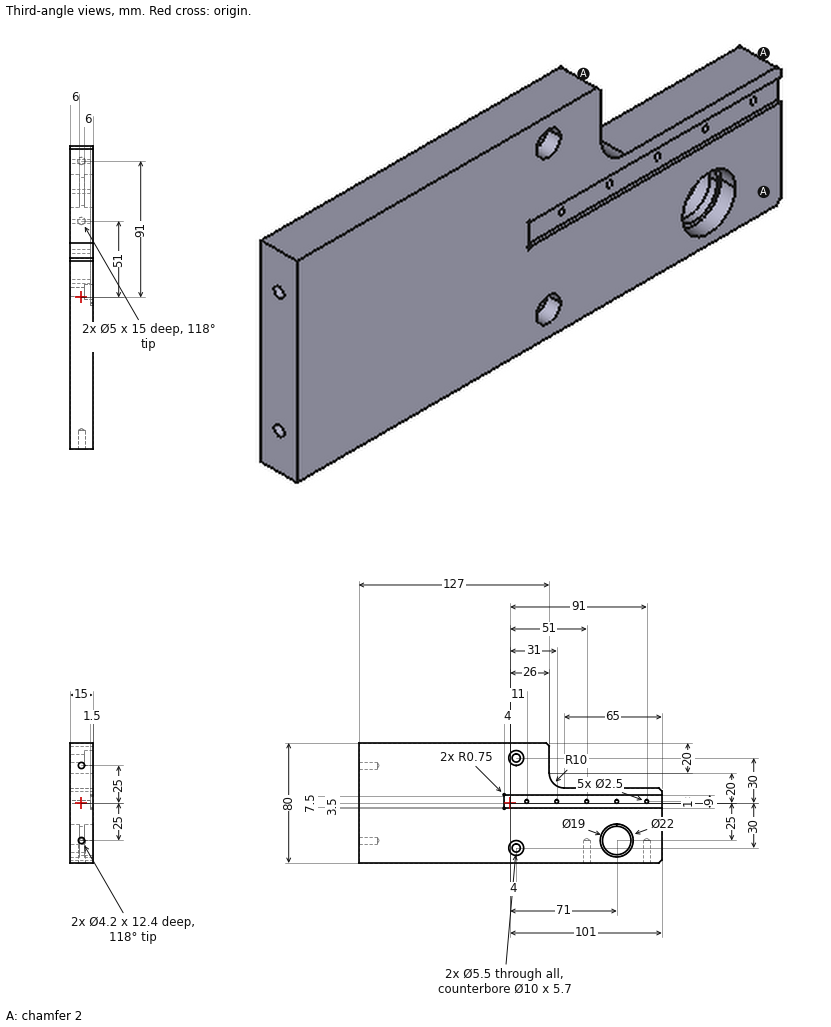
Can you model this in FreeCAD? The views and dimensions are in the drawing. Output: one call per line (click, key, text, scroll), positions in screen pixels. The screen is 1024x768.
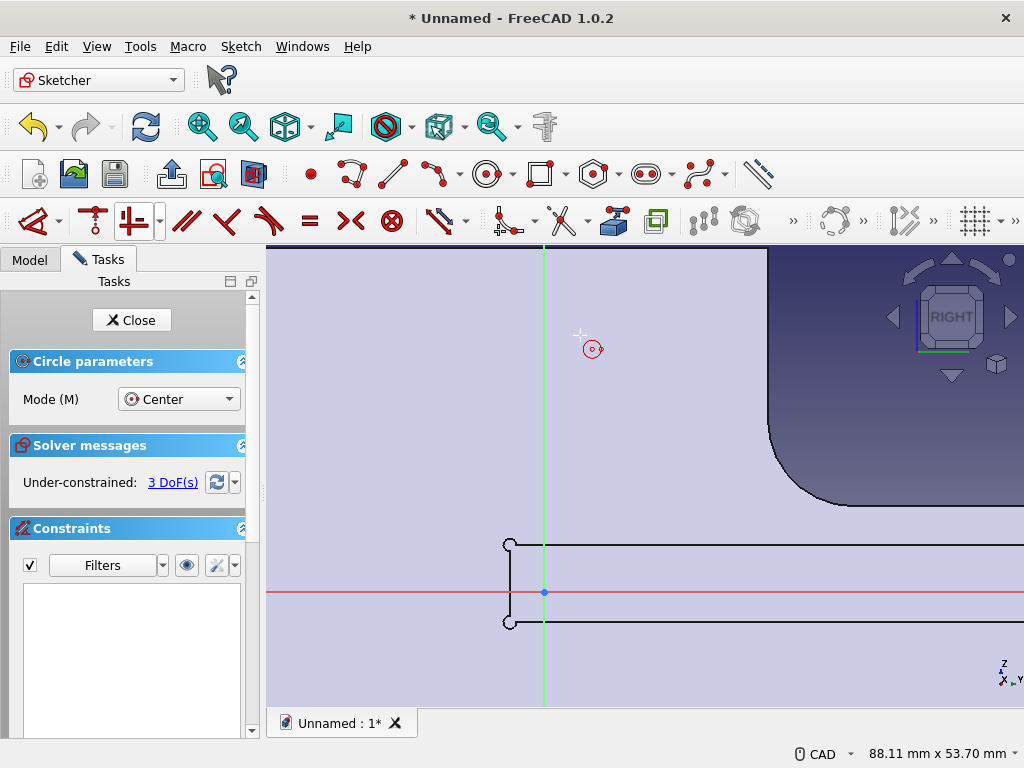
click(579, 334)
click(595, 317)
key(Escape)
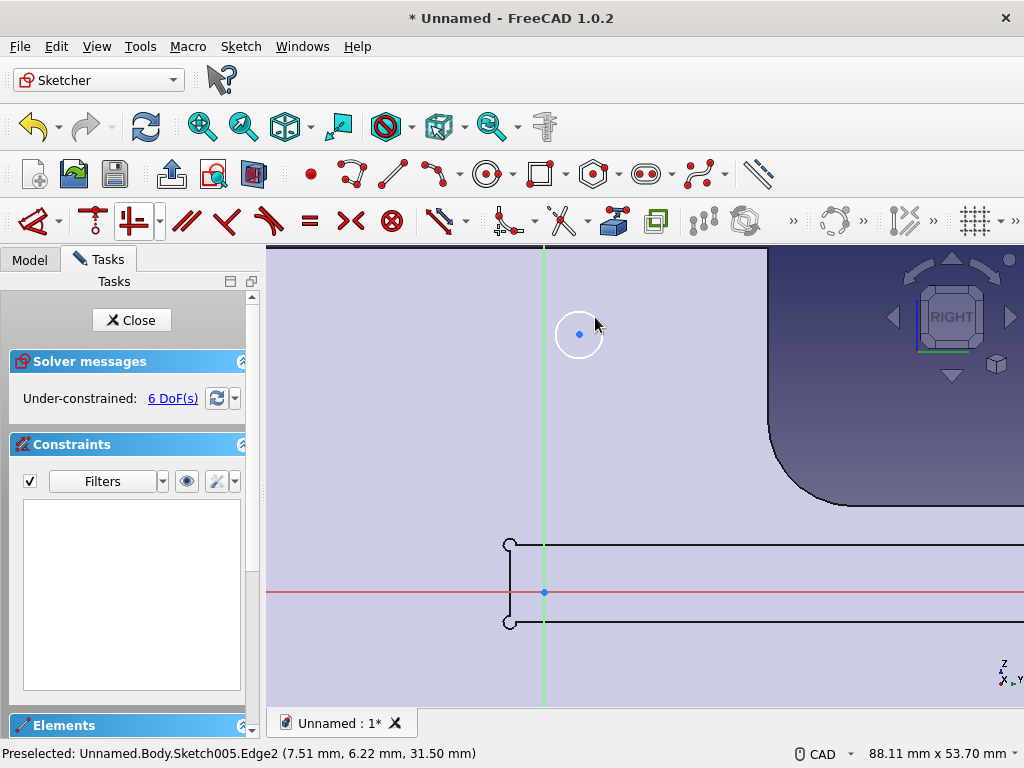
scroll(580, 335, down, 3)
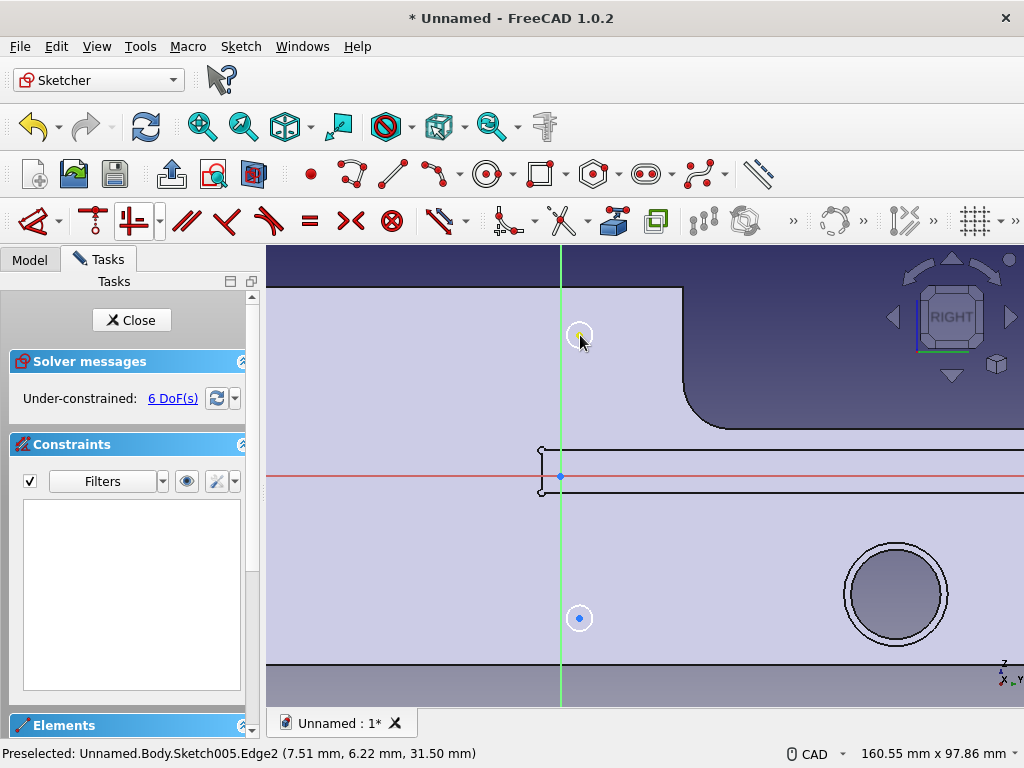
click(589, 609)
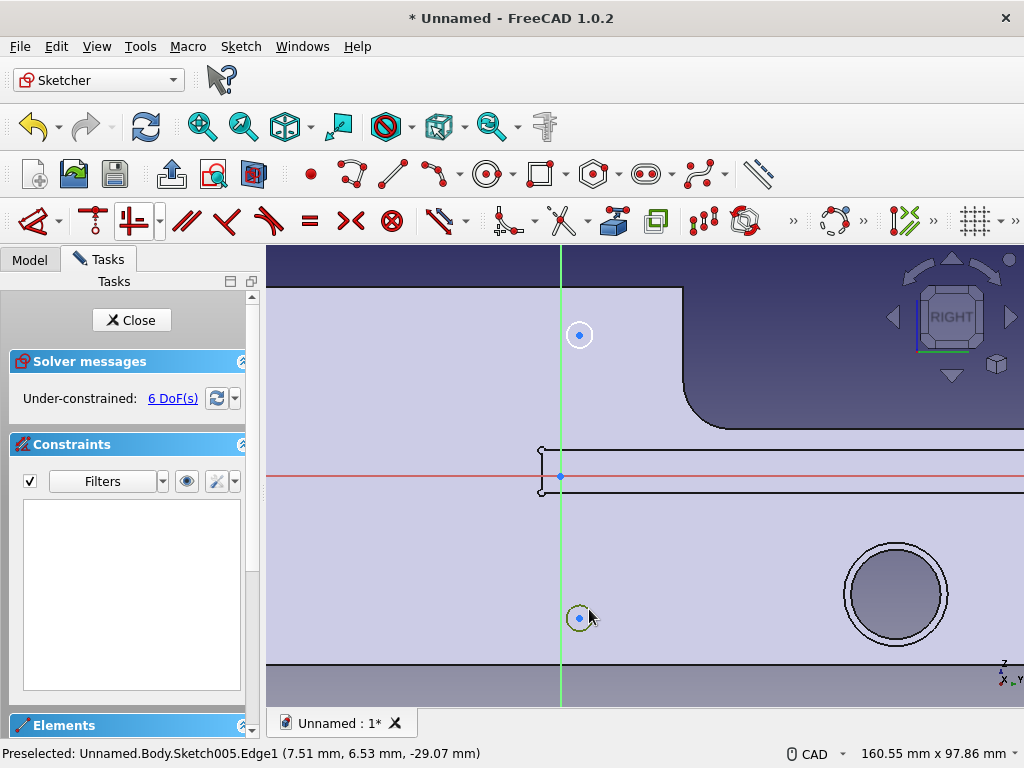
click(589, 326)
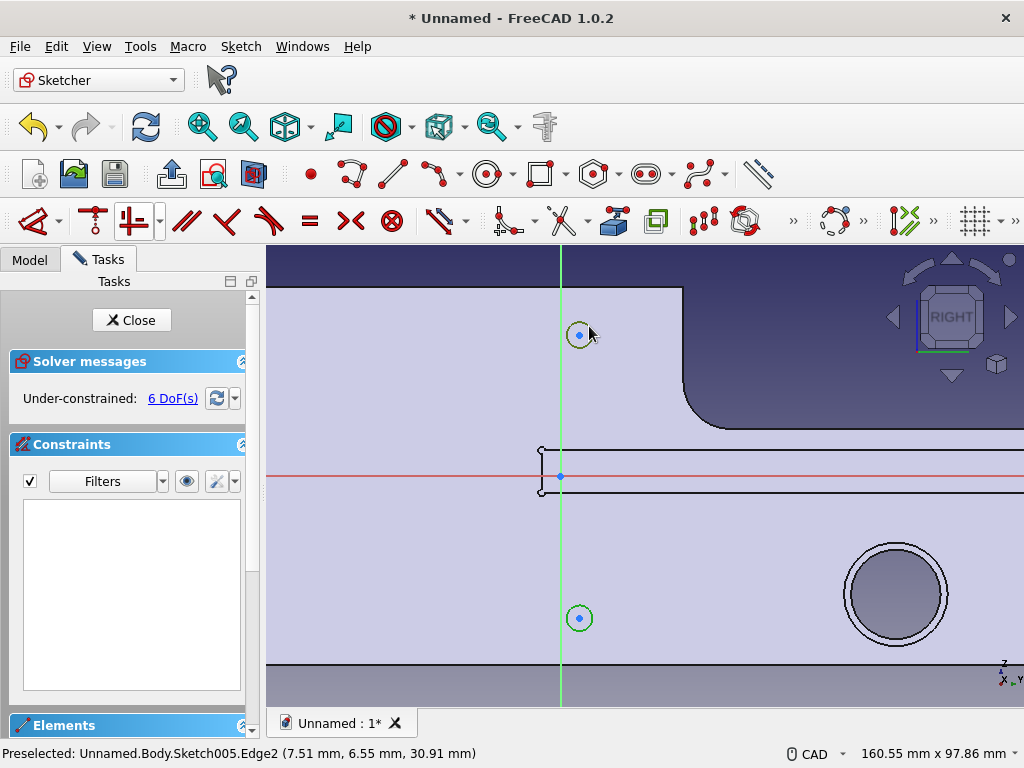
click(310, 222)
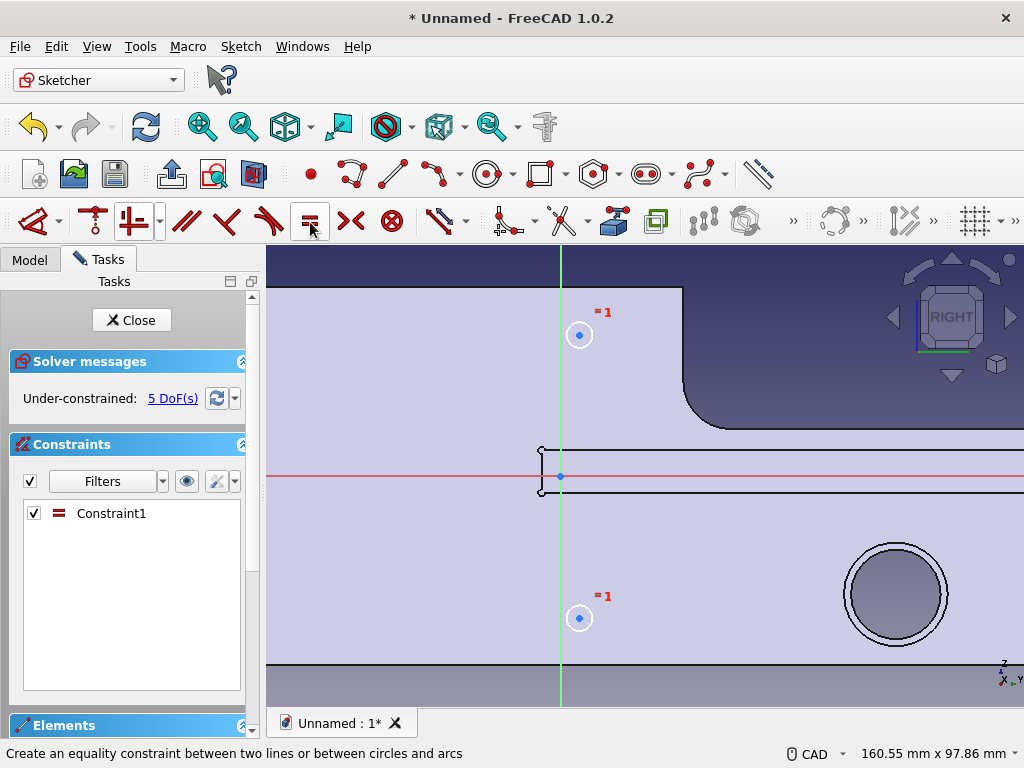
click(580, 618)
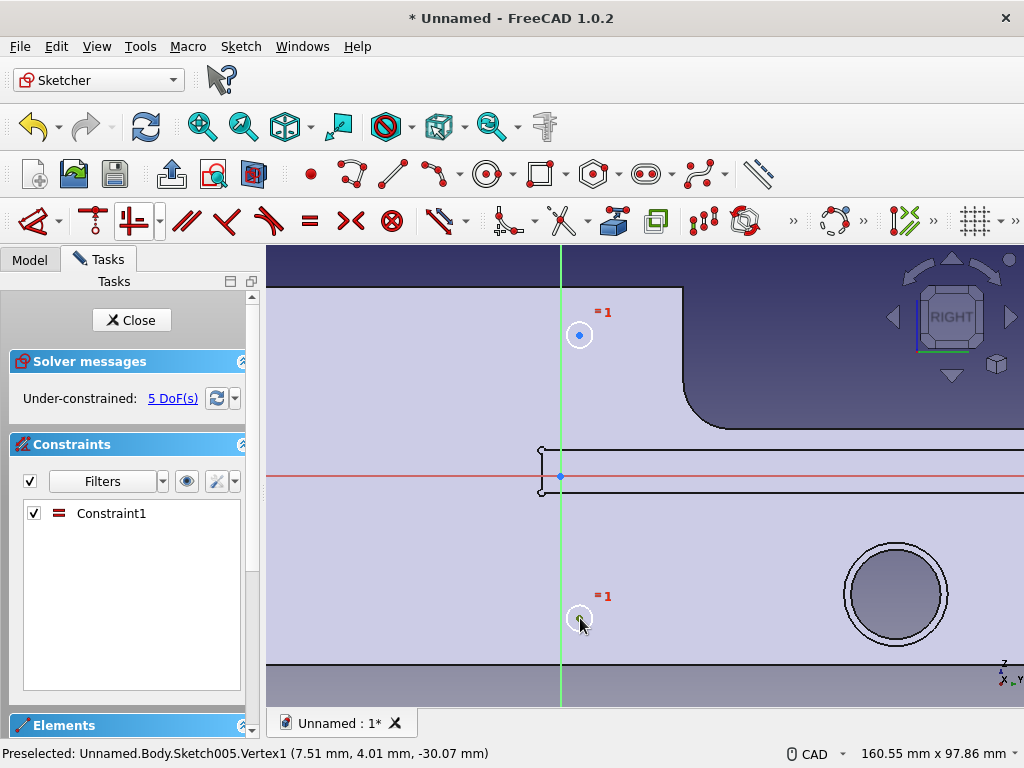
click(580, 335)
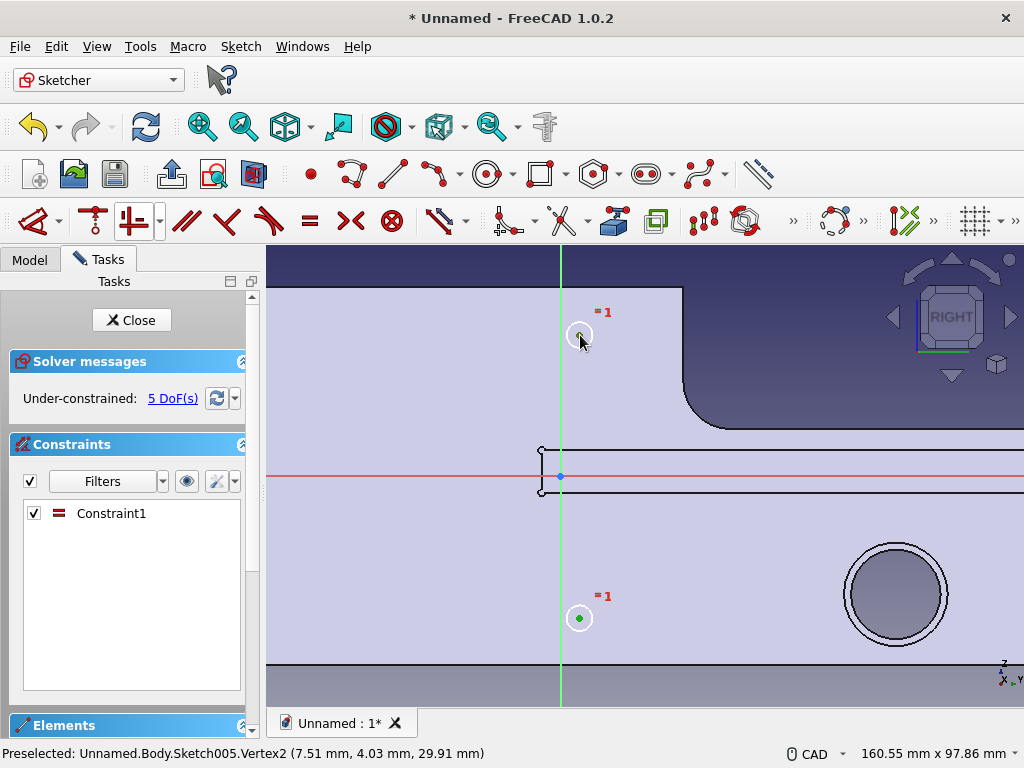
click(160, 222)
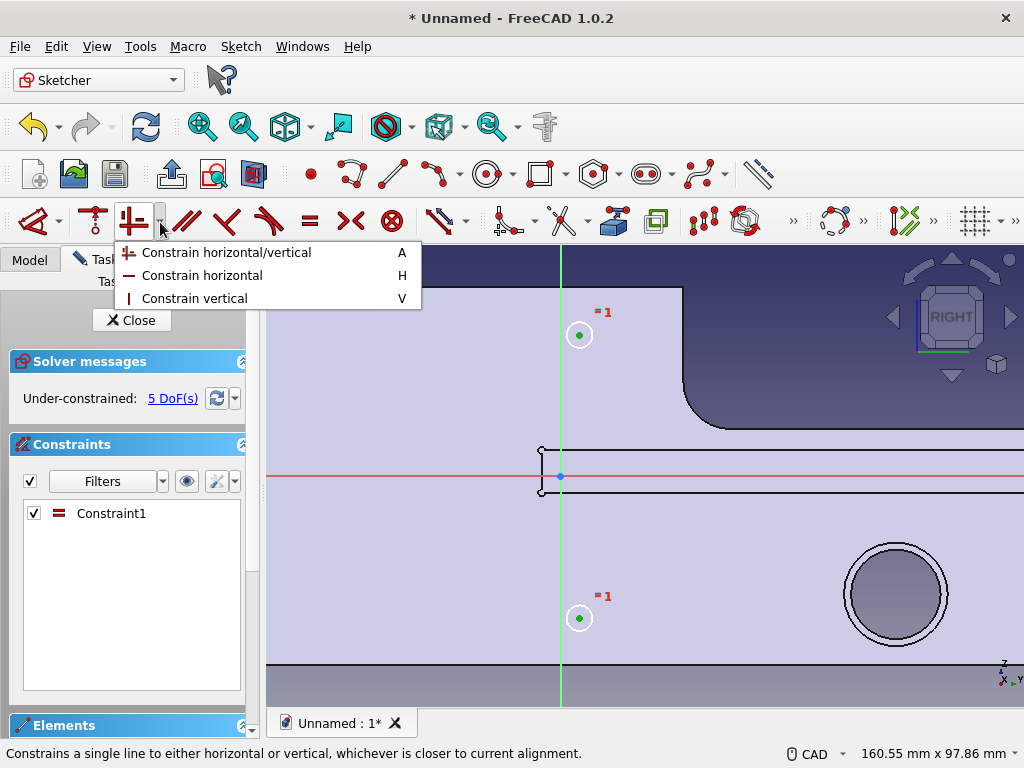
click(268, 298)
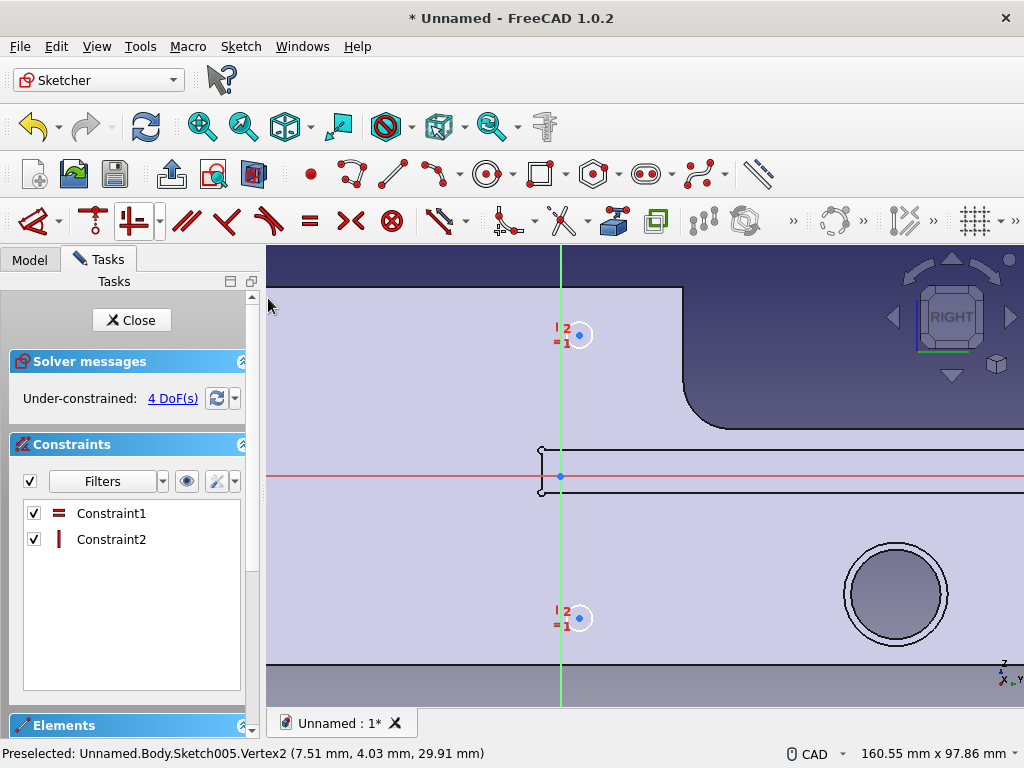
click(32, 222)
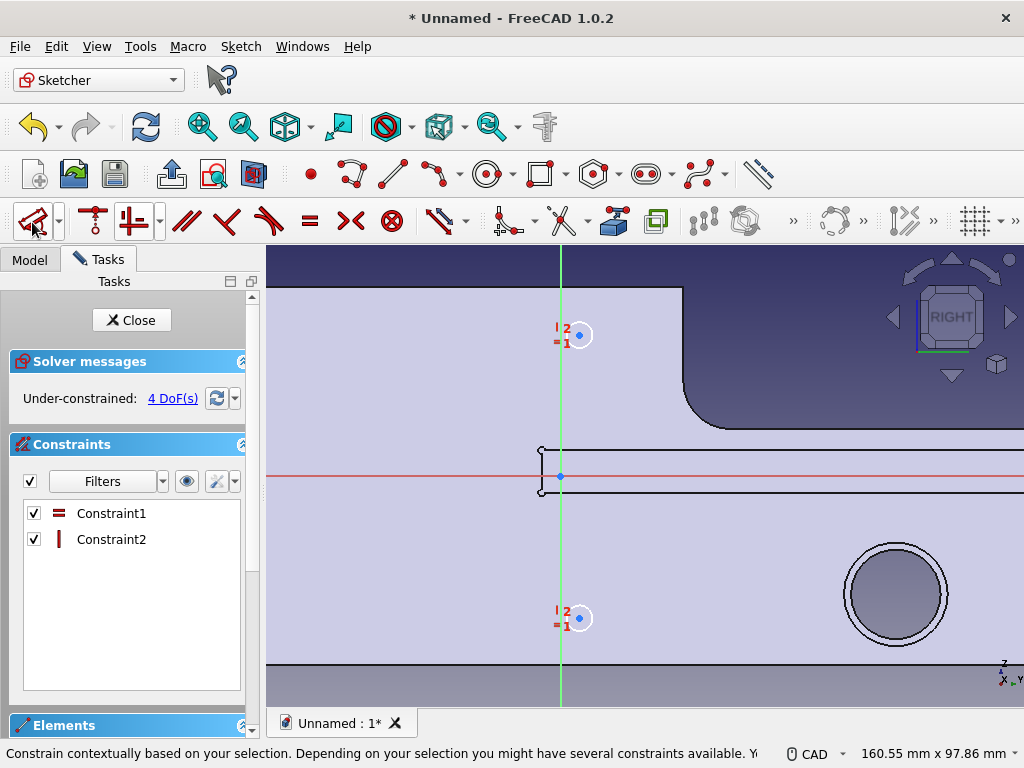
scroll(589, 609, up, 3)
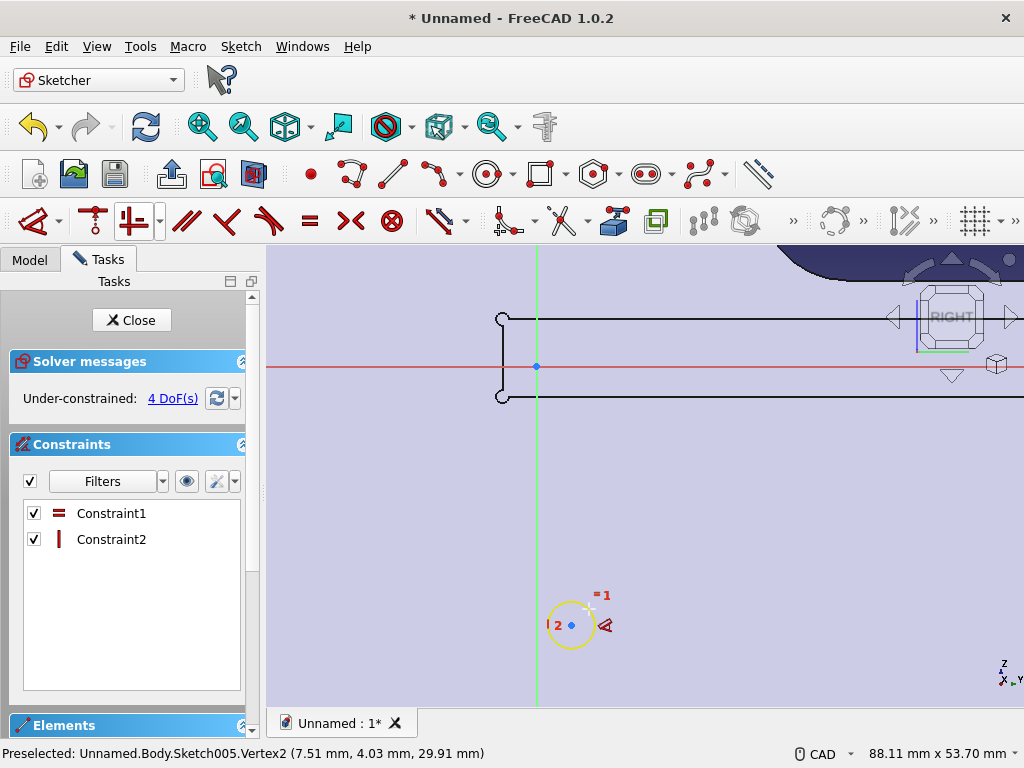
click(588, 609)
click(611, 587)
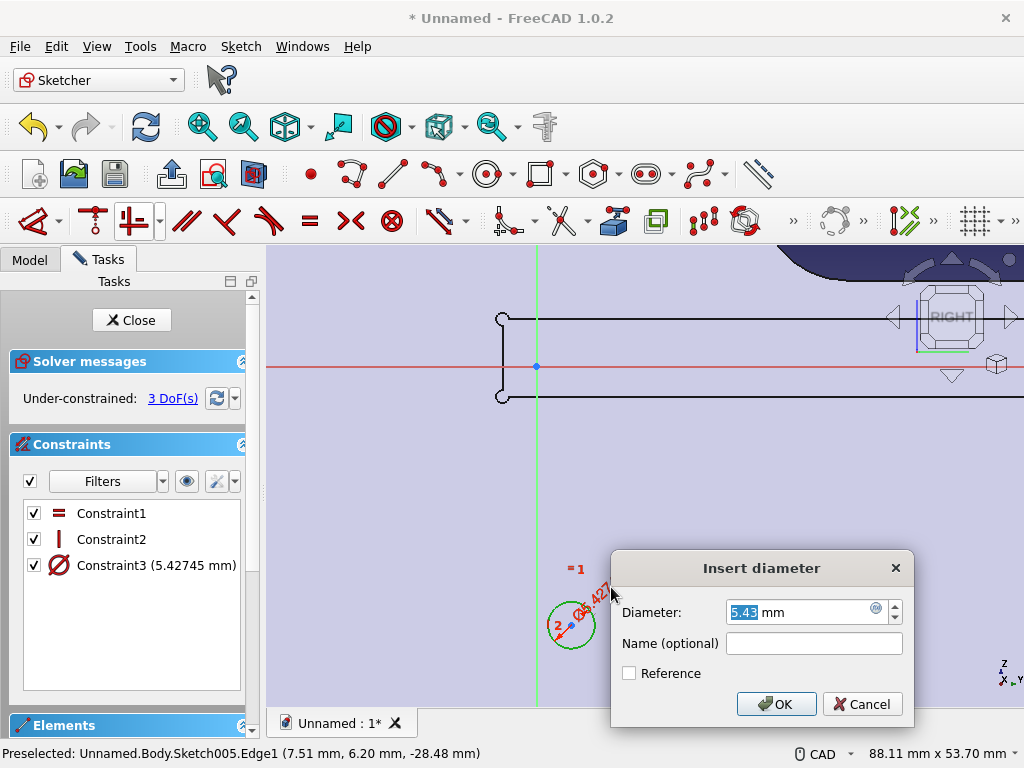
text(5.5)
key(Return)